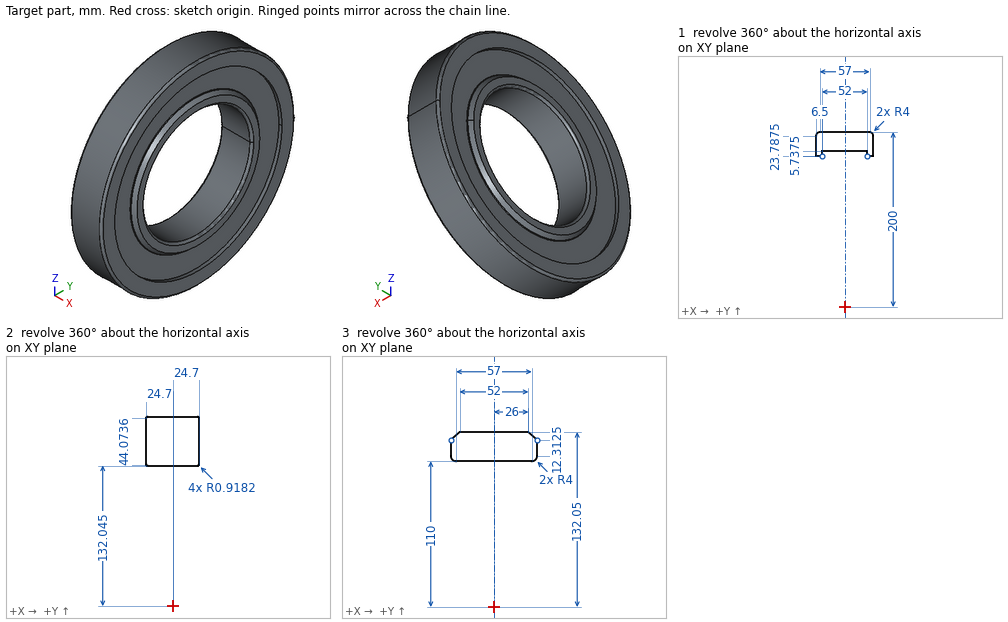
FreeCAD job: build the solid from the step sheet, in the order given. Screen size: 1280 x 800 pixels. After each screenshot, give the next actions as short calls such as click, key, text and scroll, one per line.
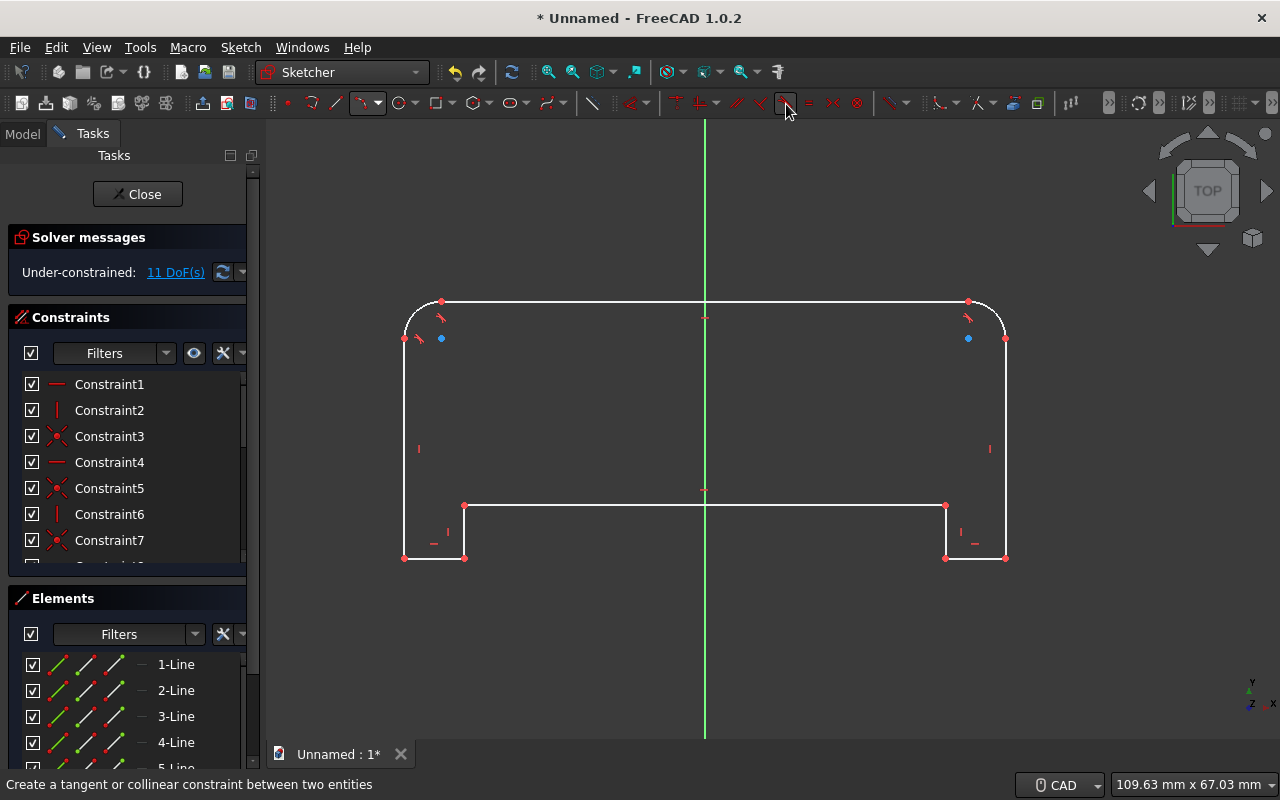
click(1006, 493)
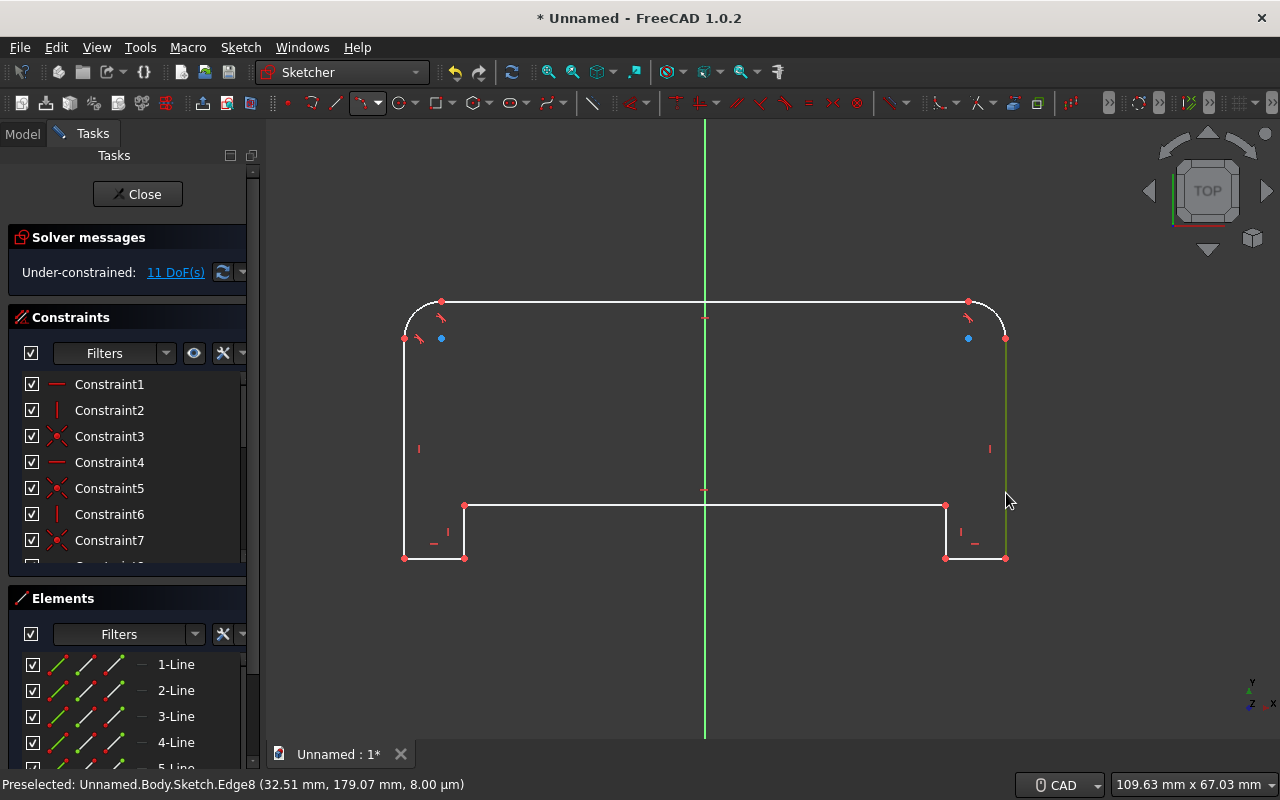
click(1002, 322)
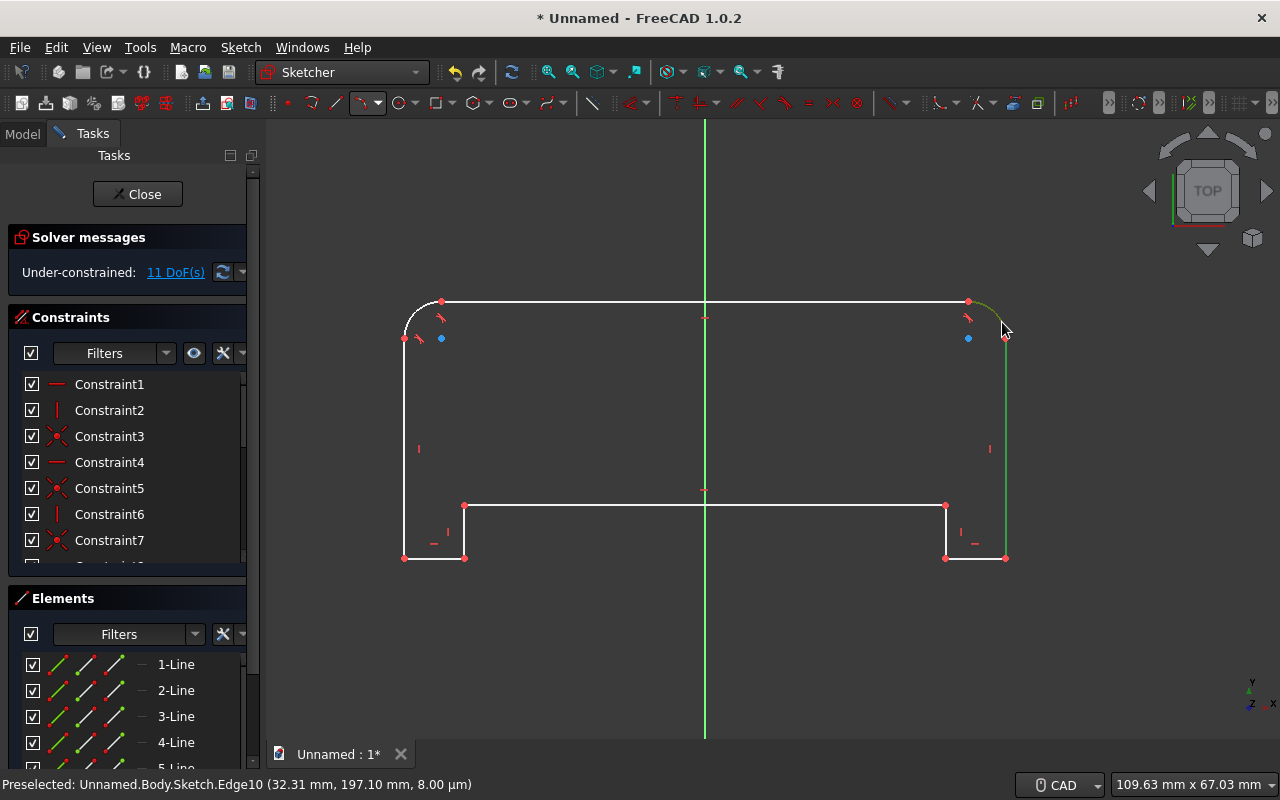
click(786, 104)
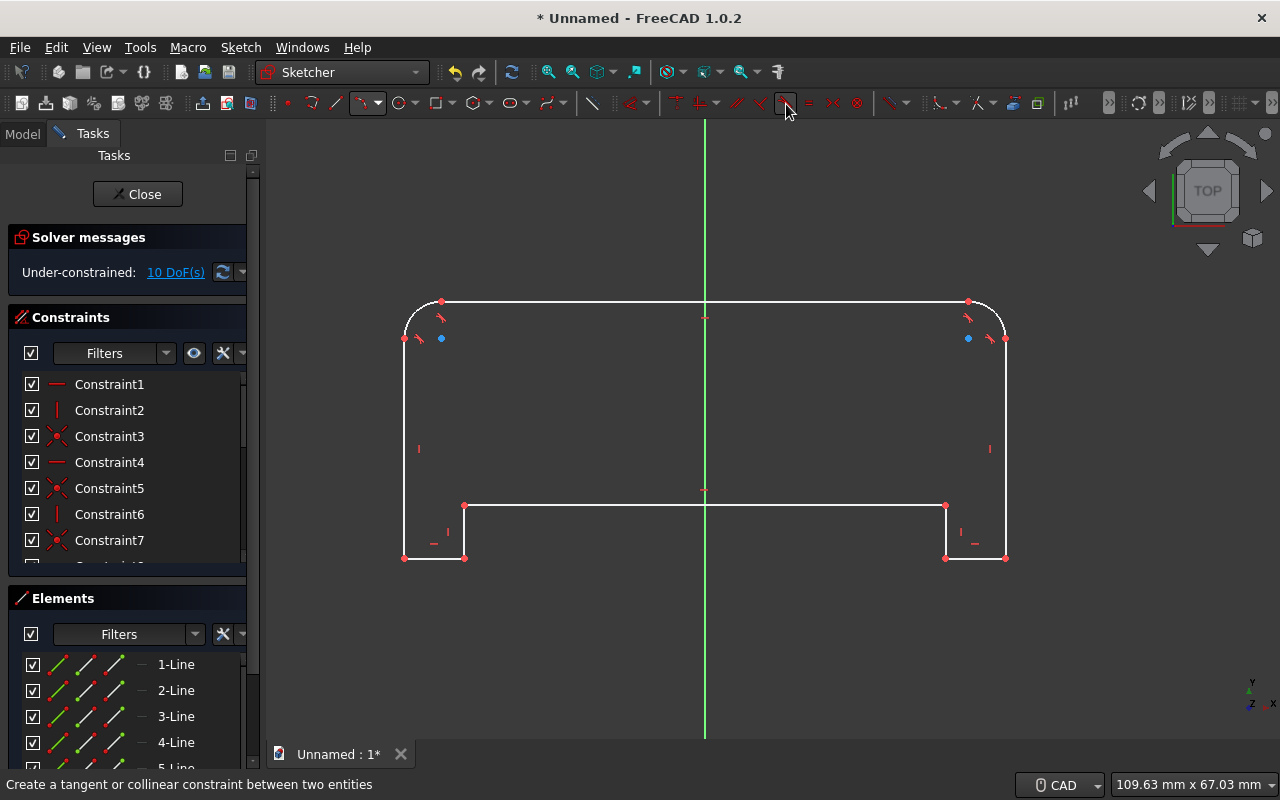
click(425, 306)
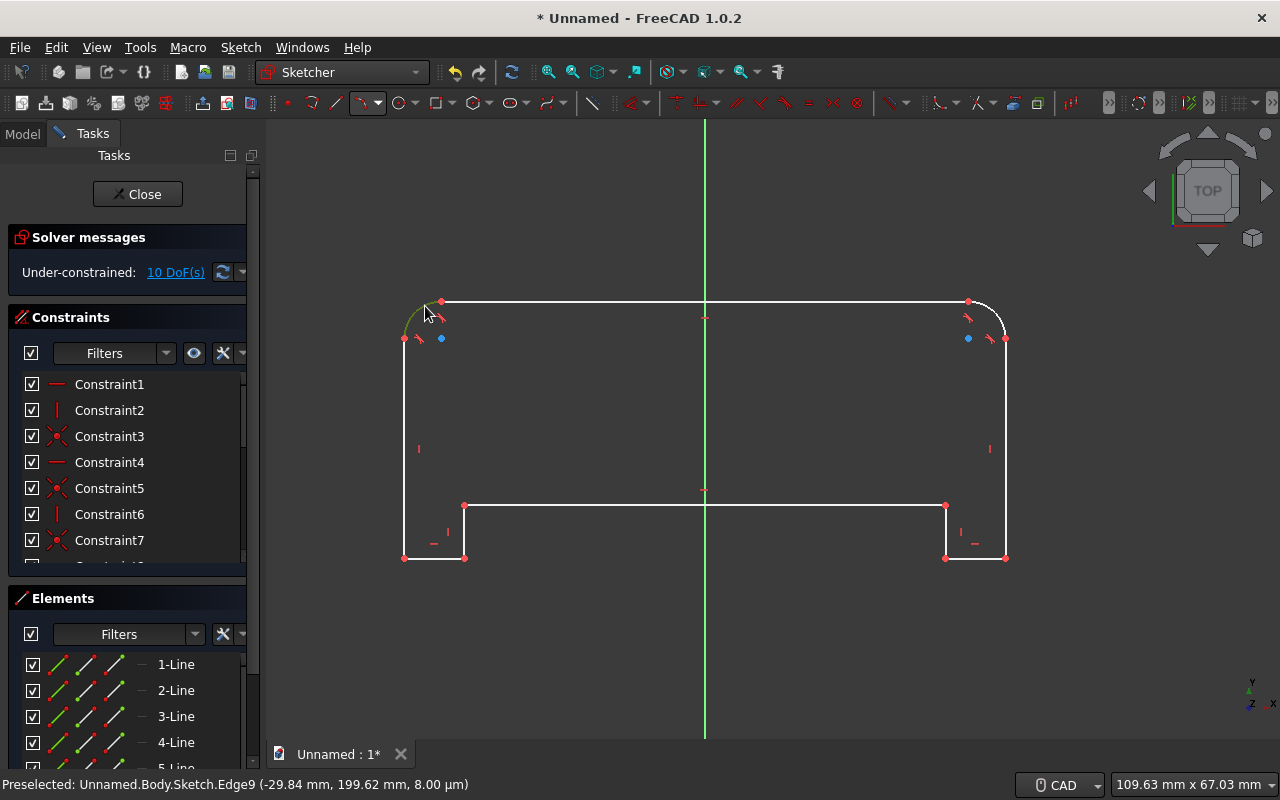
click(1002, 322)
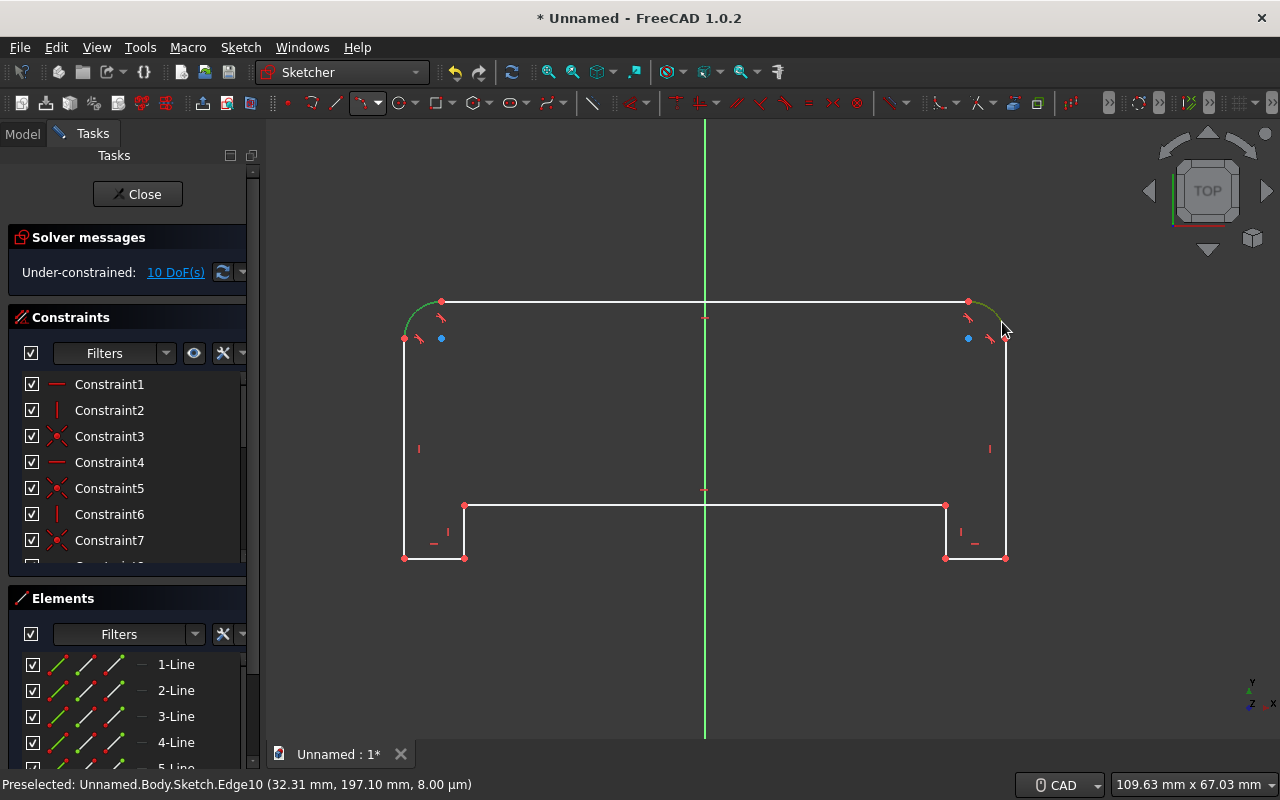
click(810, 104)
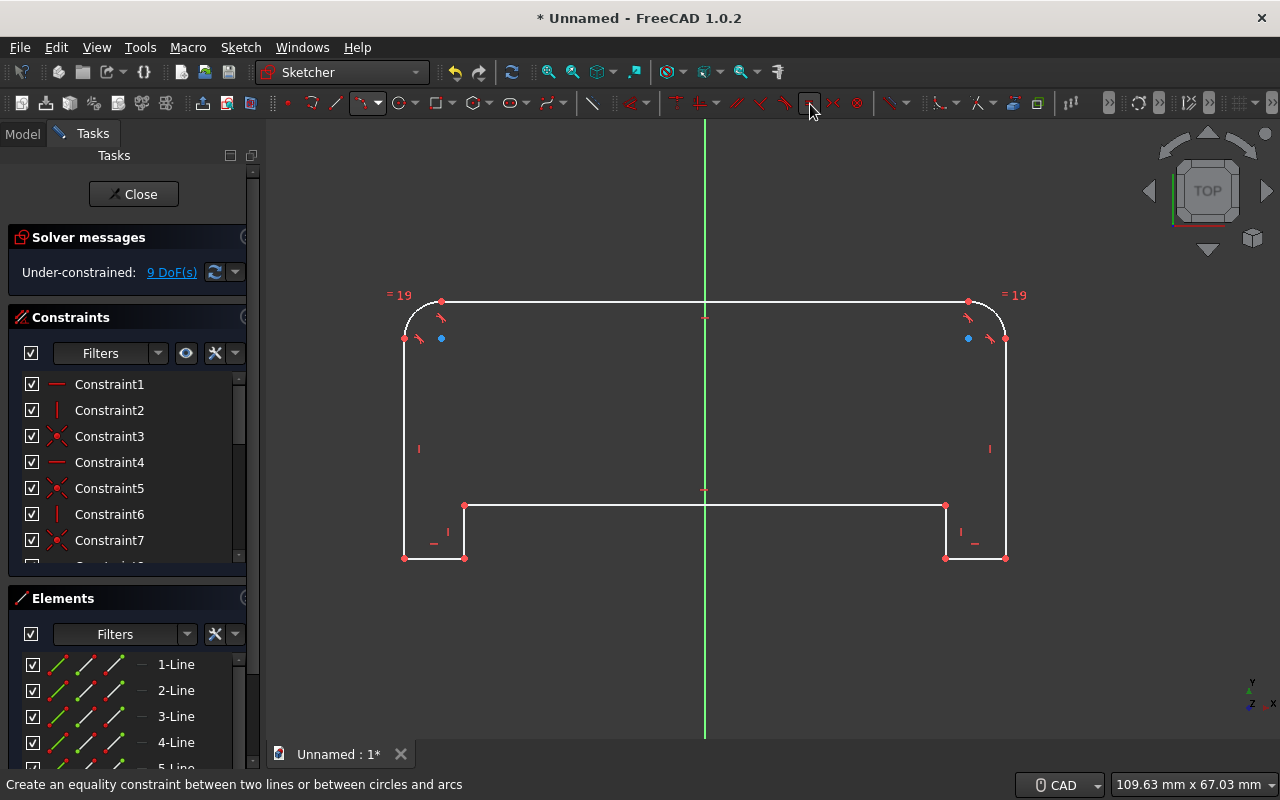
click(464, 559)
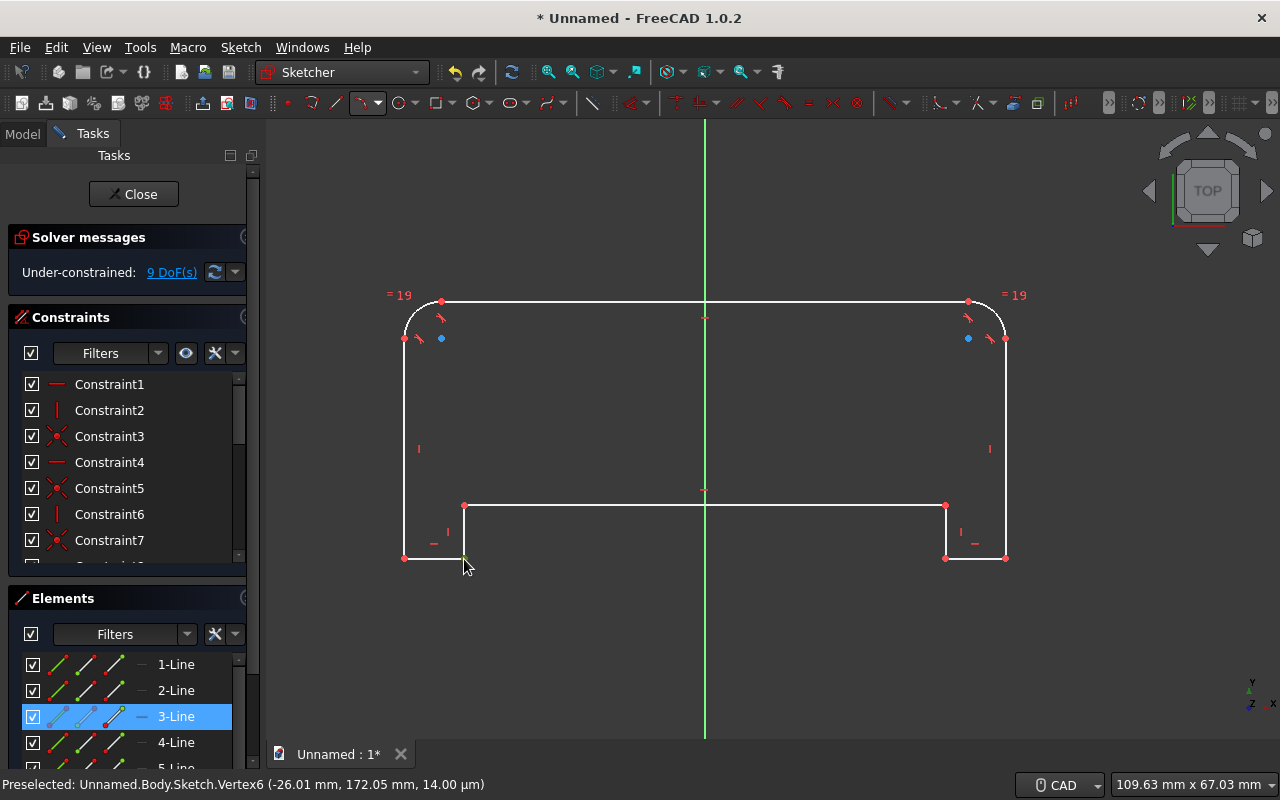
click(946, 559)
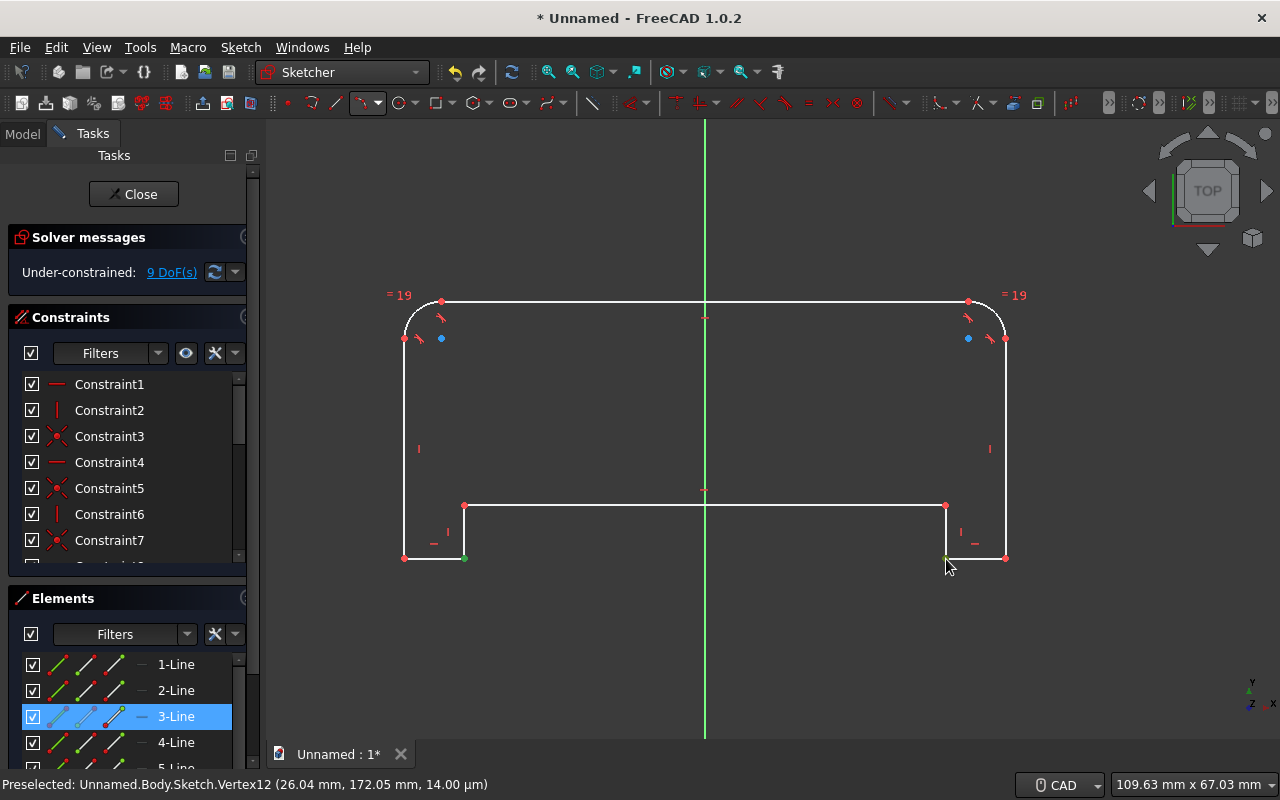
click(705, 671)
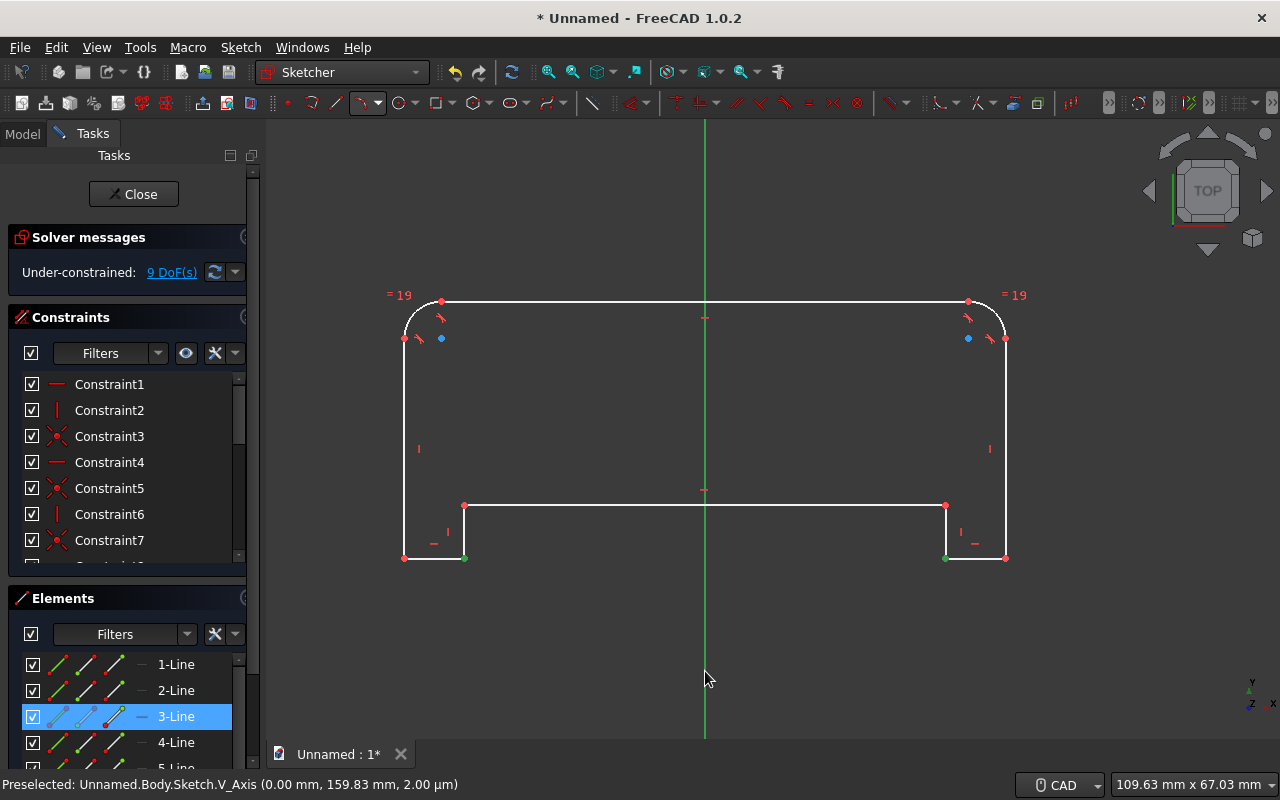
click(834, 104)